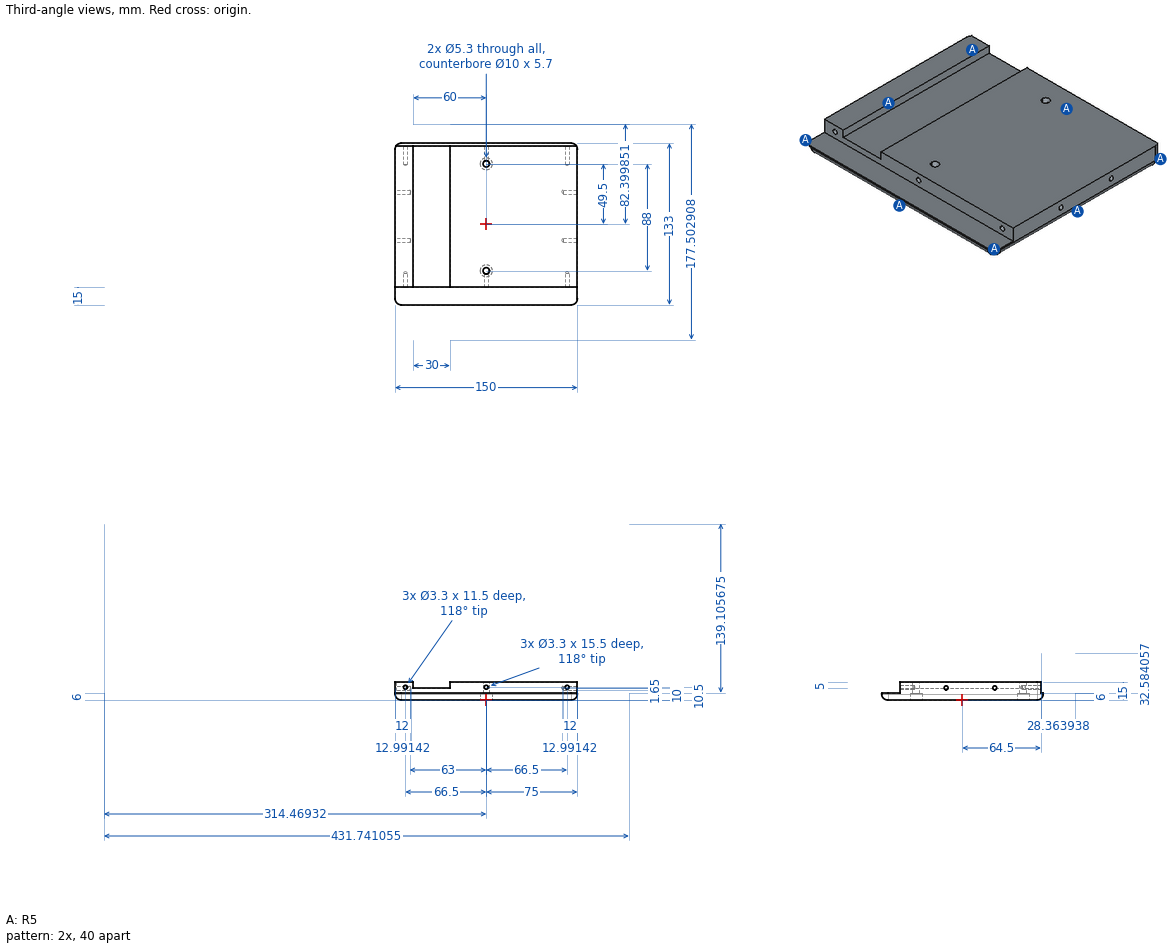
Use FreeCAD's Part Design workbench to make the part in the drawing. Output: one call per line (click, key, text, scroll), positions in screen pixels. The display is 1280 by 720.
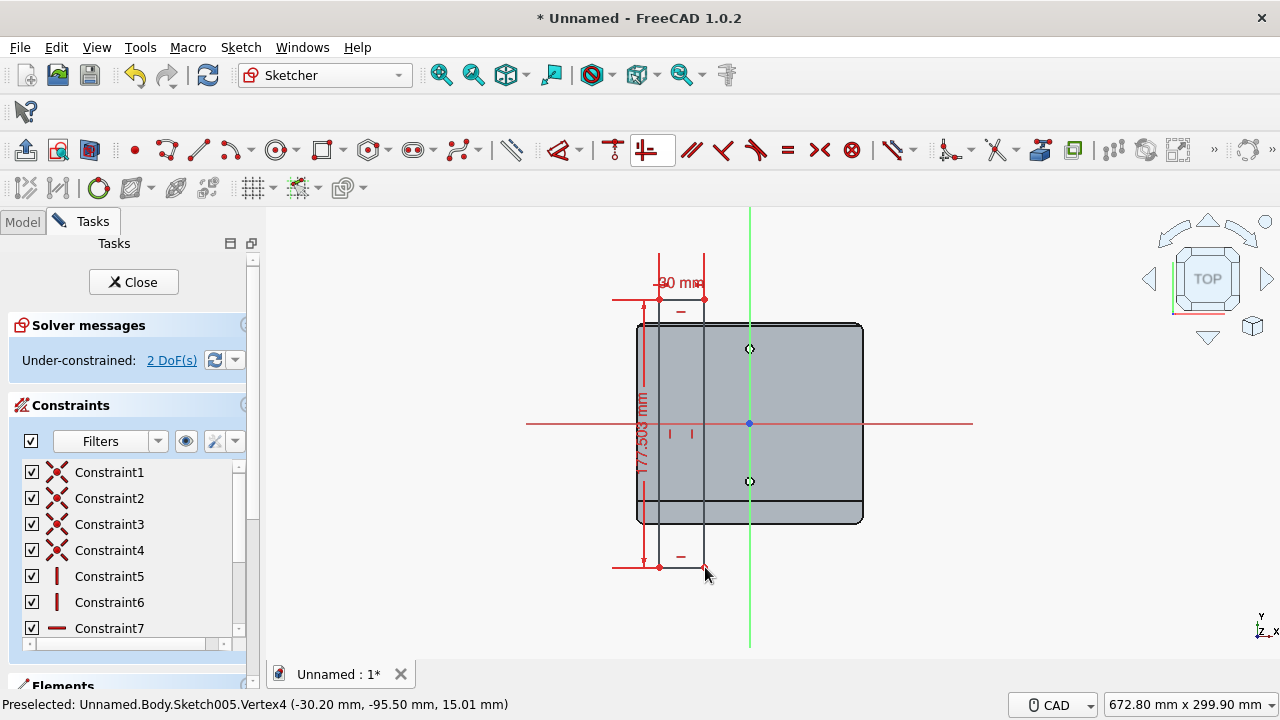
click(558, 150)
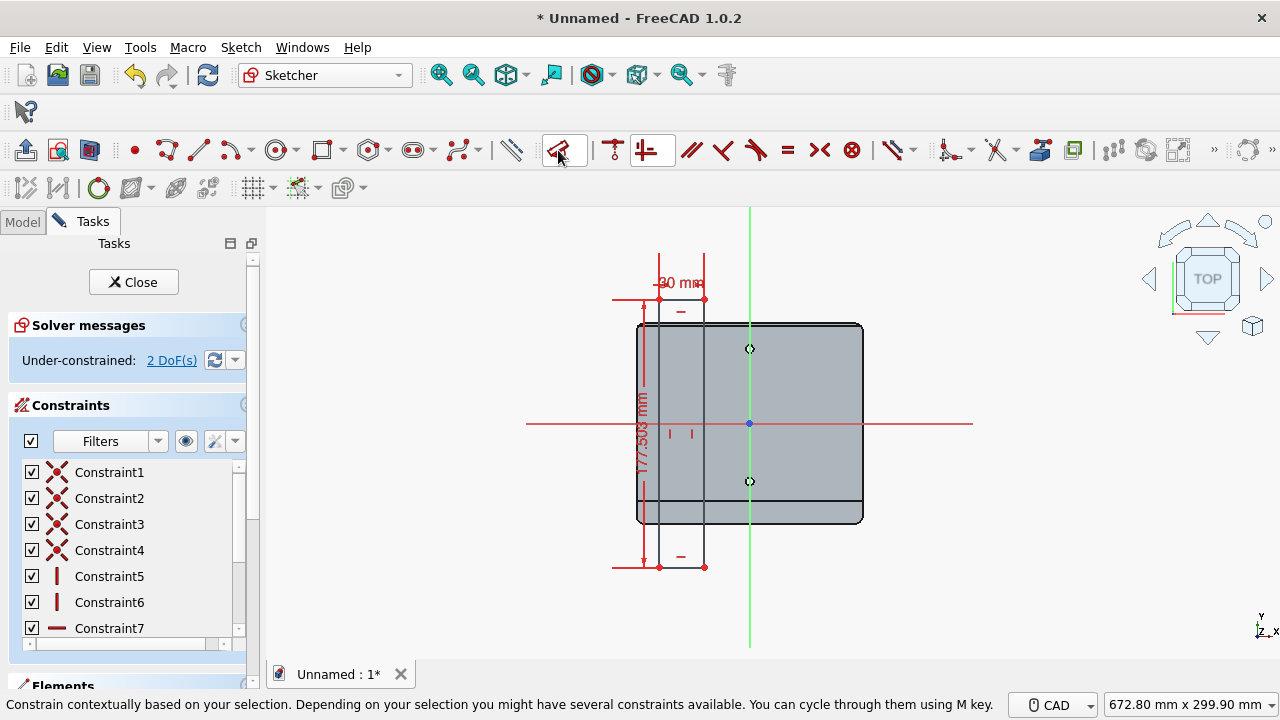
click(659, 300)
click(704, 266)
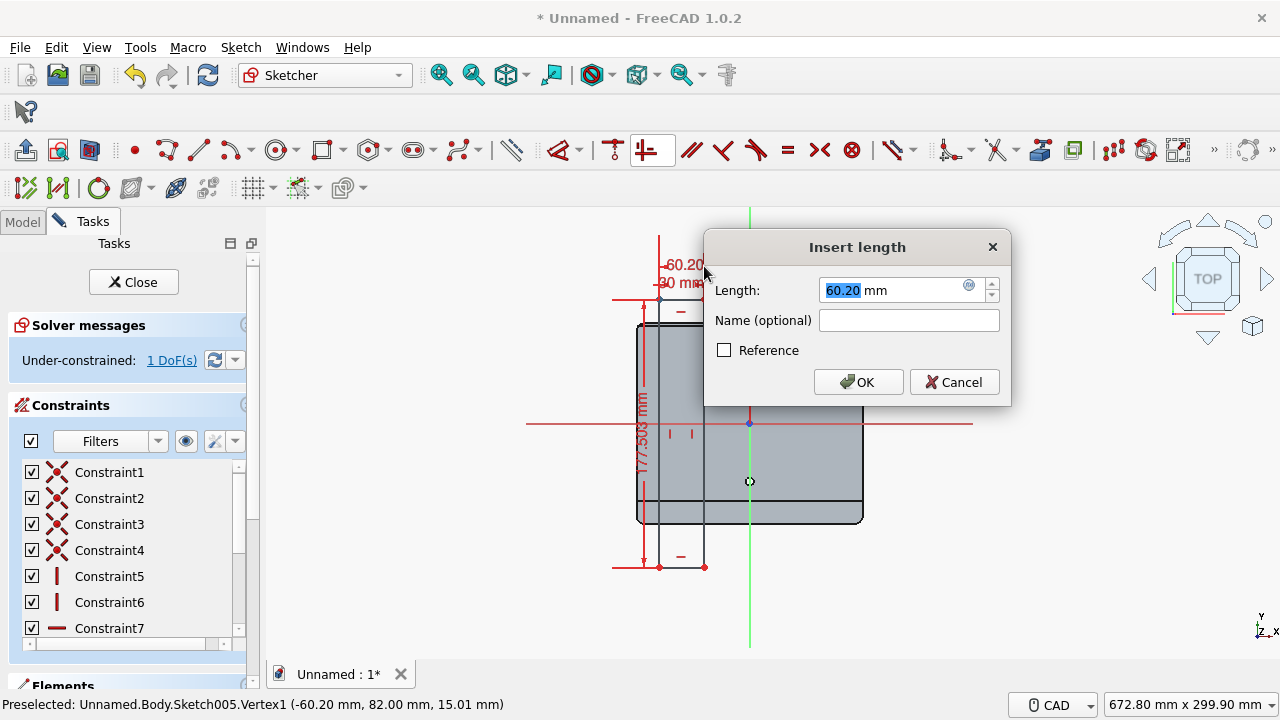
text(60)
key(Return)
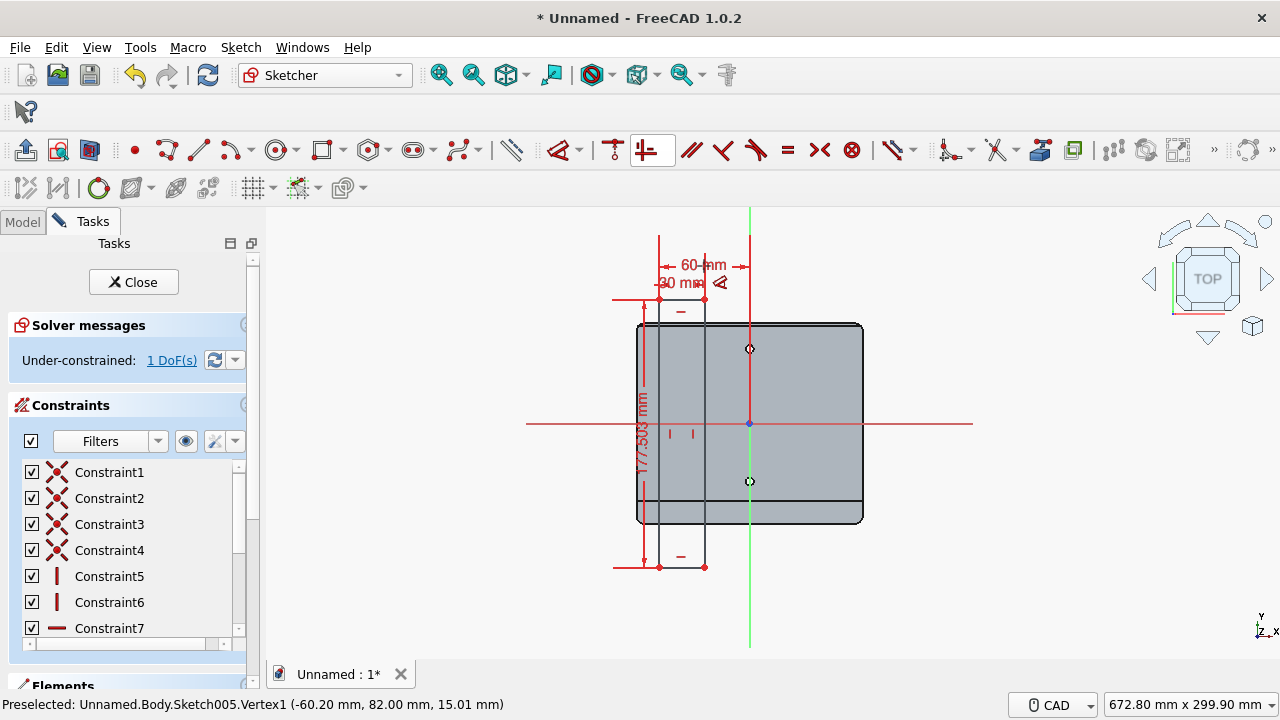
click(659, 300)
click(784, 362)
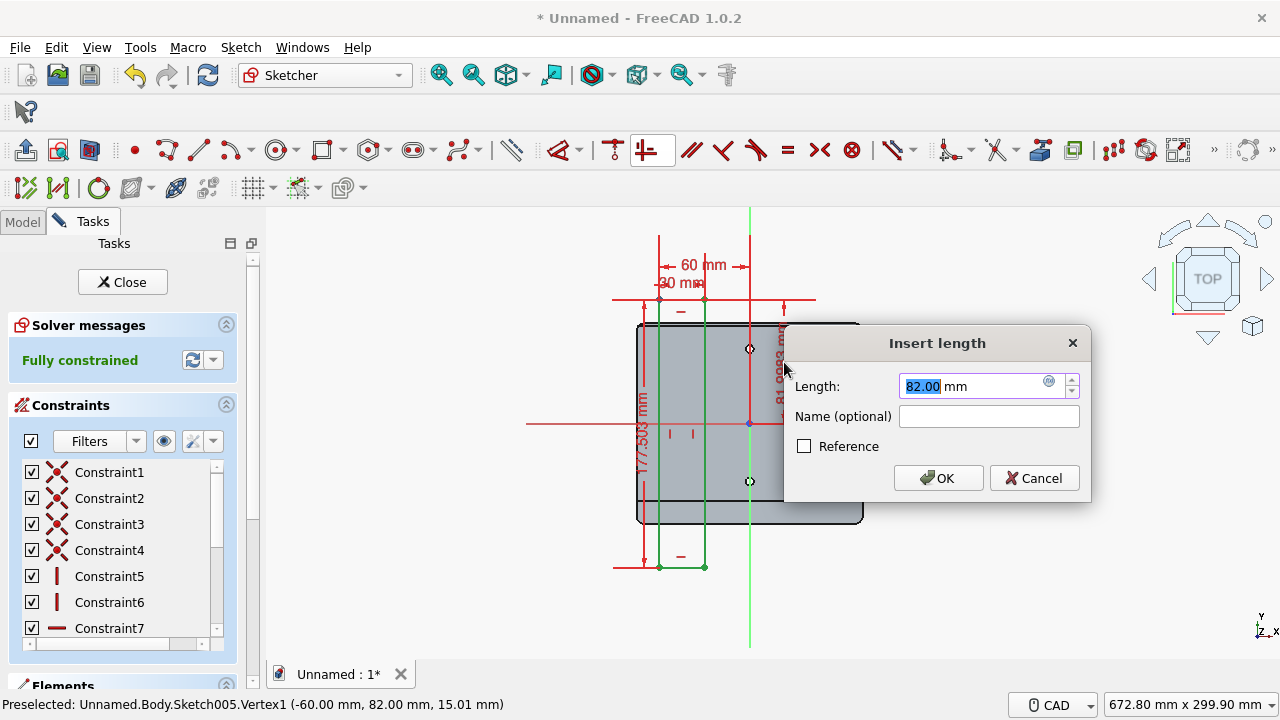
text(82.399851)
key(Return)
key(Escape)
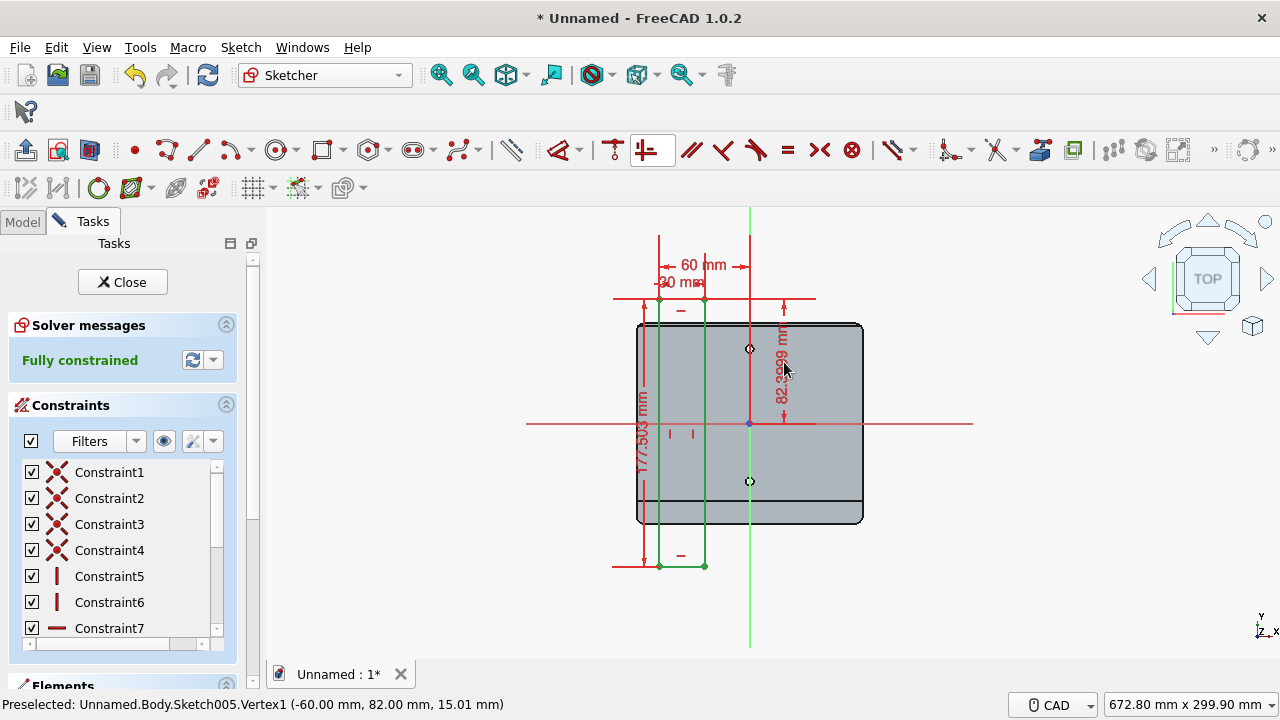
click(123, 282)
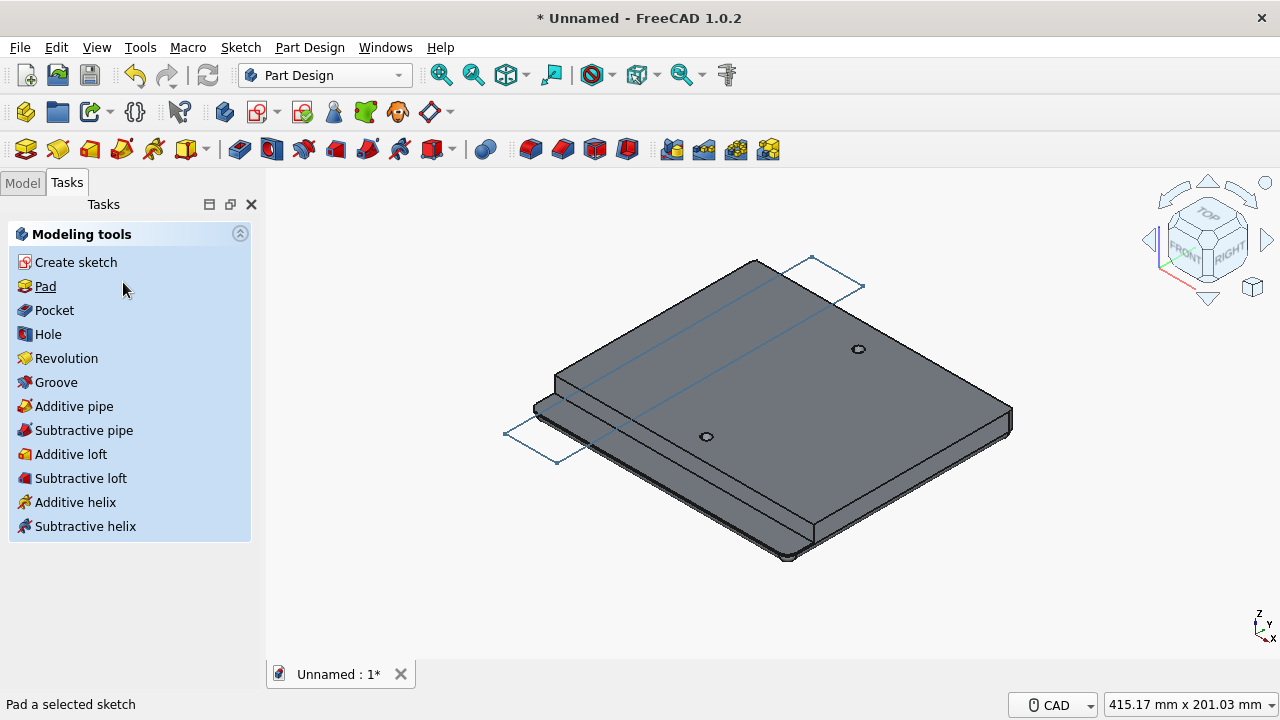
click(240, 150)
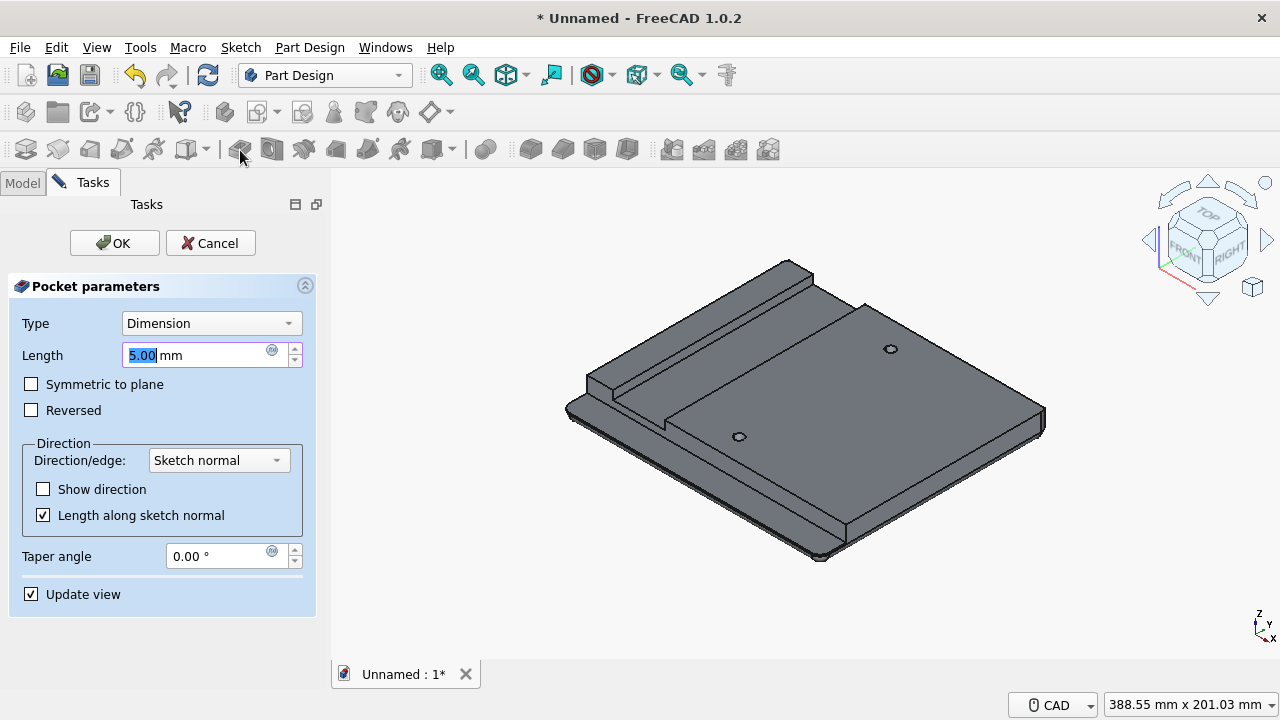
text(5)
key(Tab)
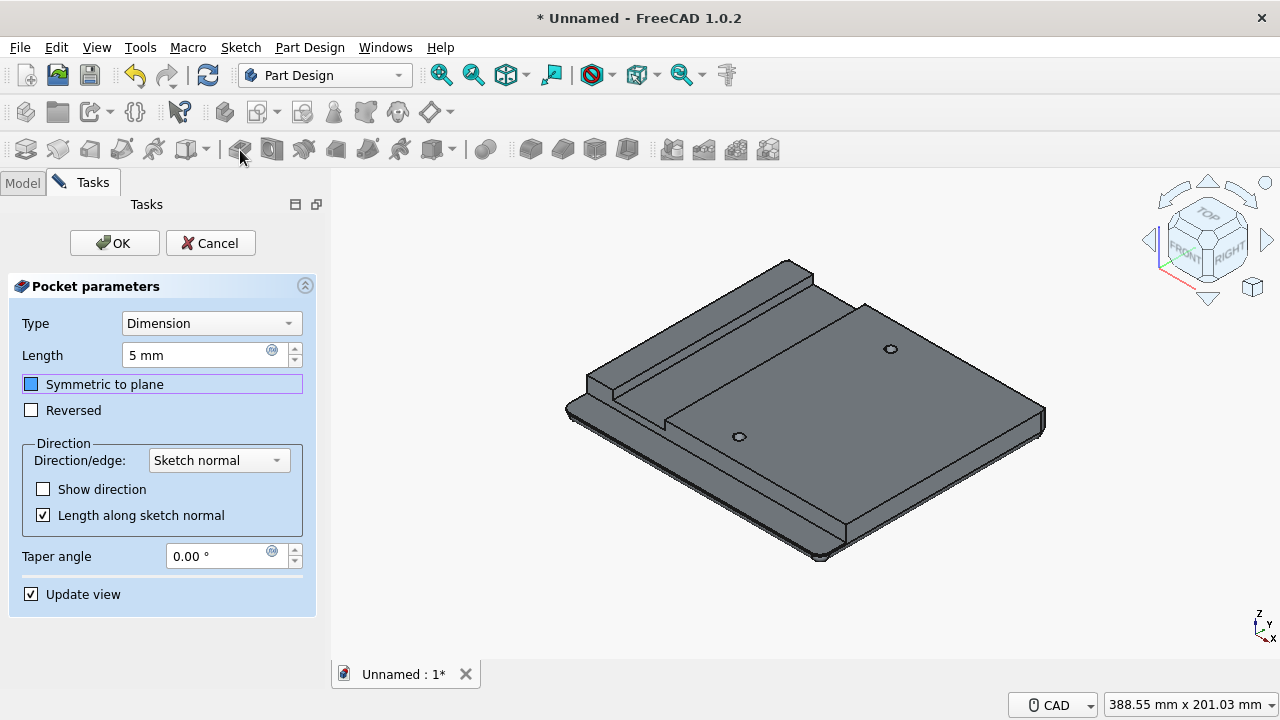
click(115, 243)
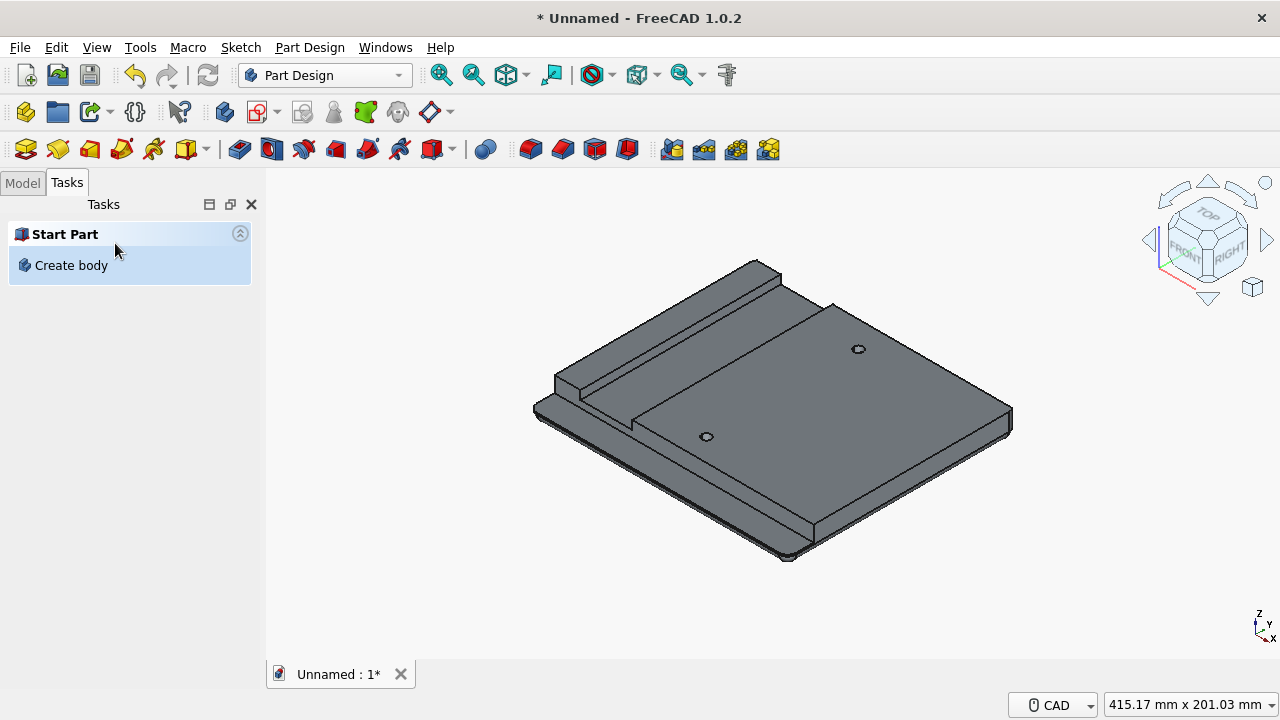
key(1)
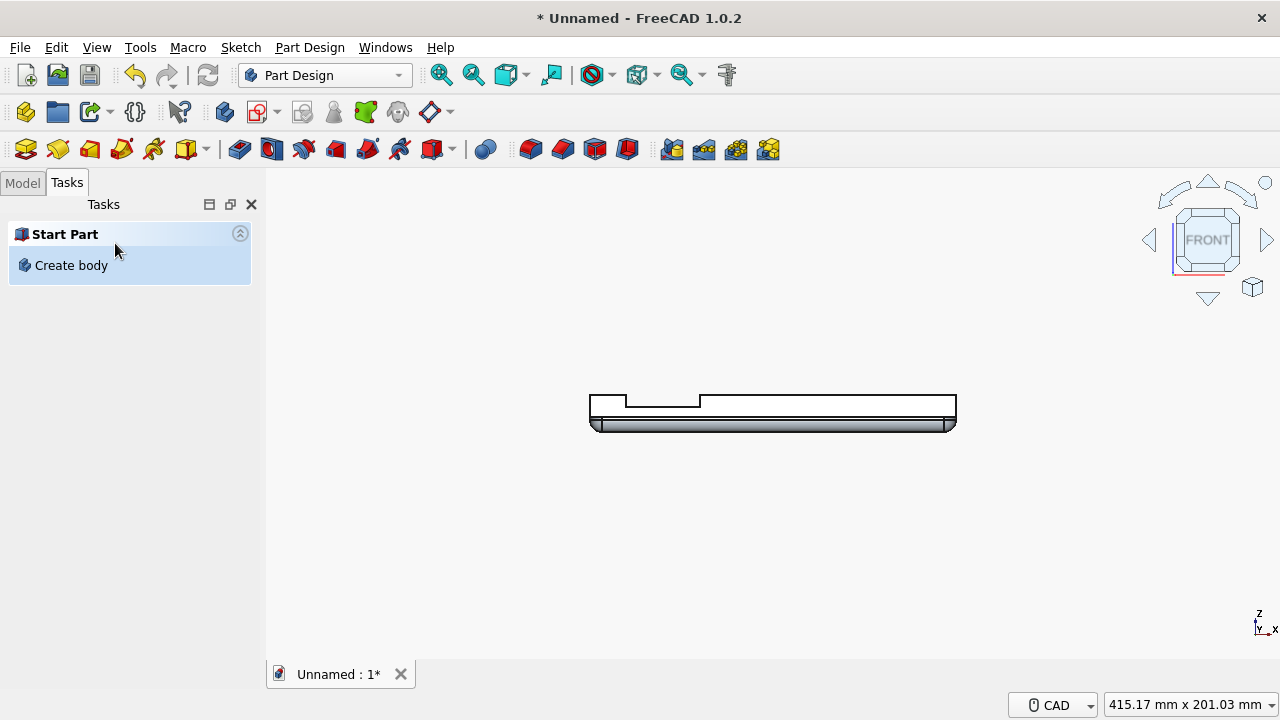
click(442, 76)